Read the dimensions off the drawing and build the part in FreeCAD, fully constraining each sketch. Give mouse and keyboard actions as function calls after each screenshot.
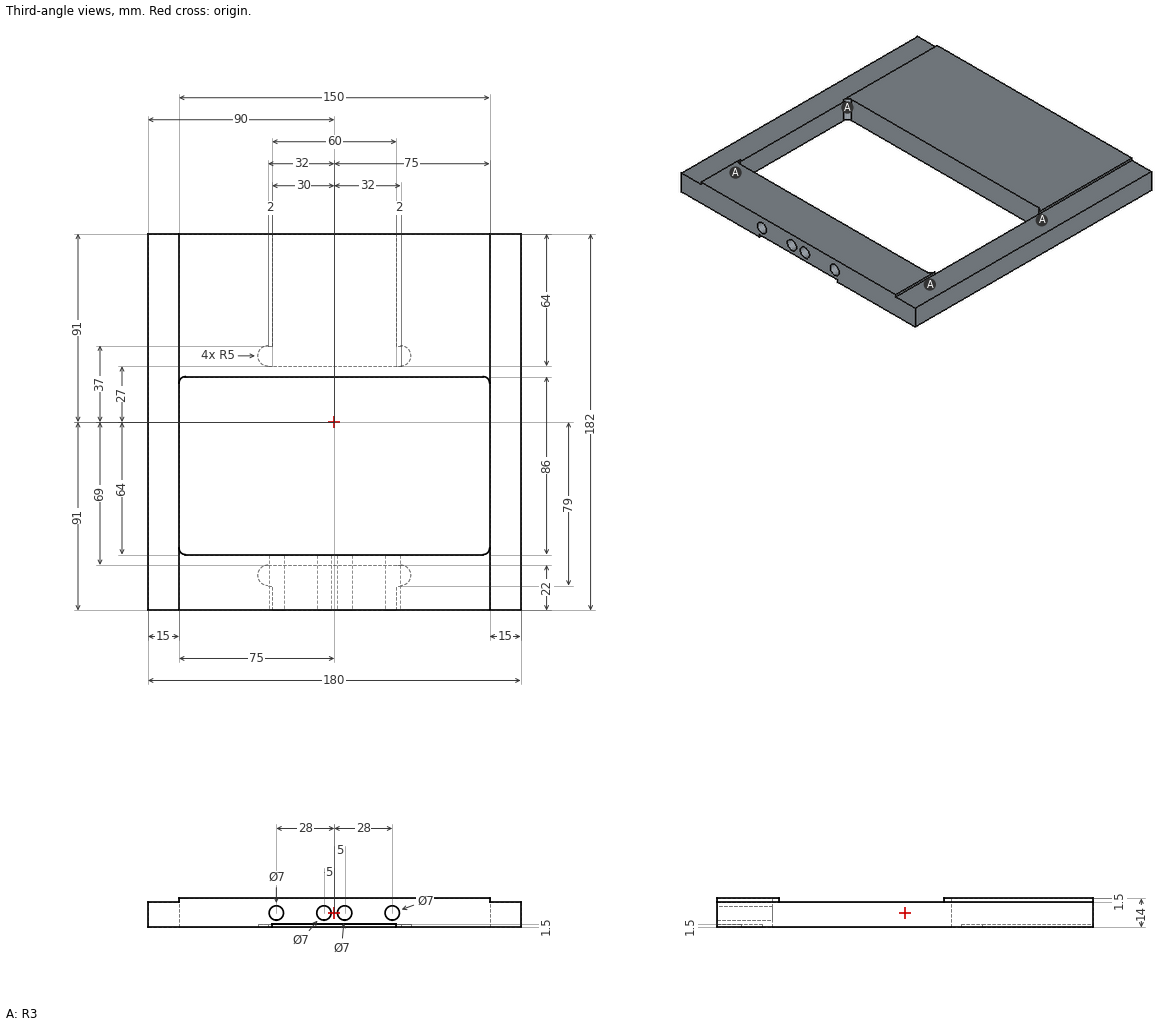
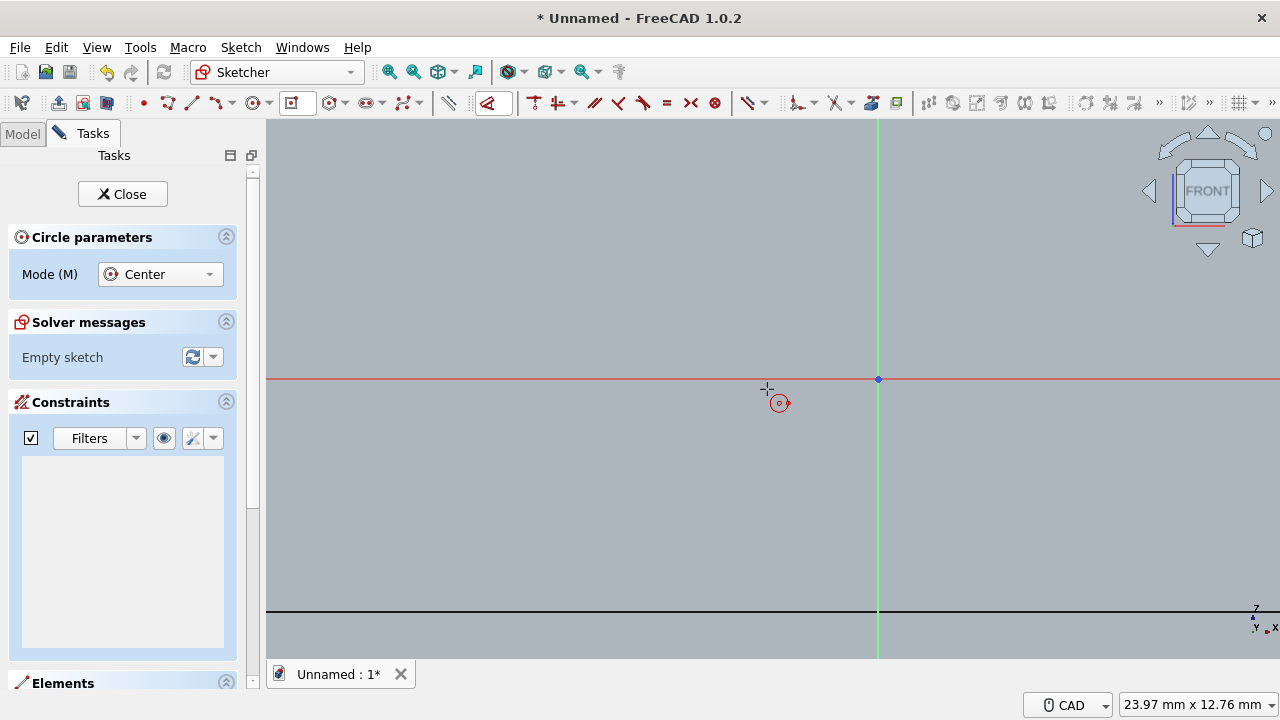
click(667, 379)
move(771, 275)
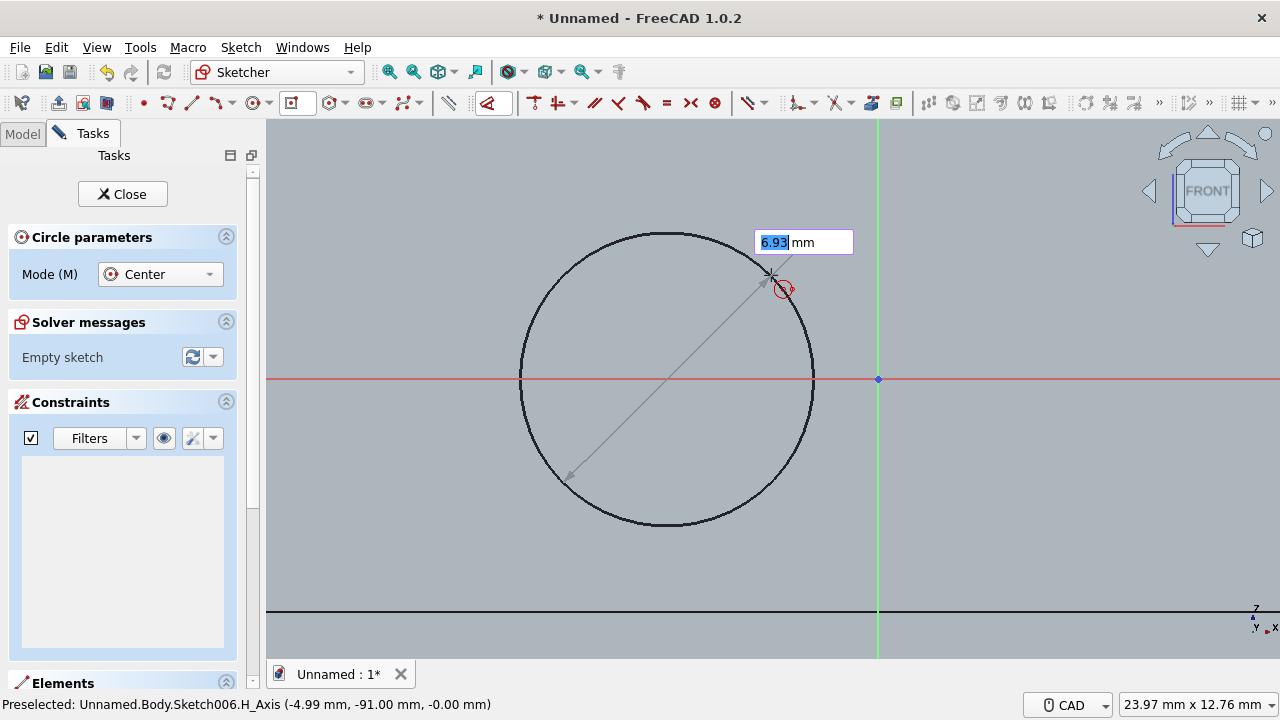
text(7)
key(Return)
key(Escape)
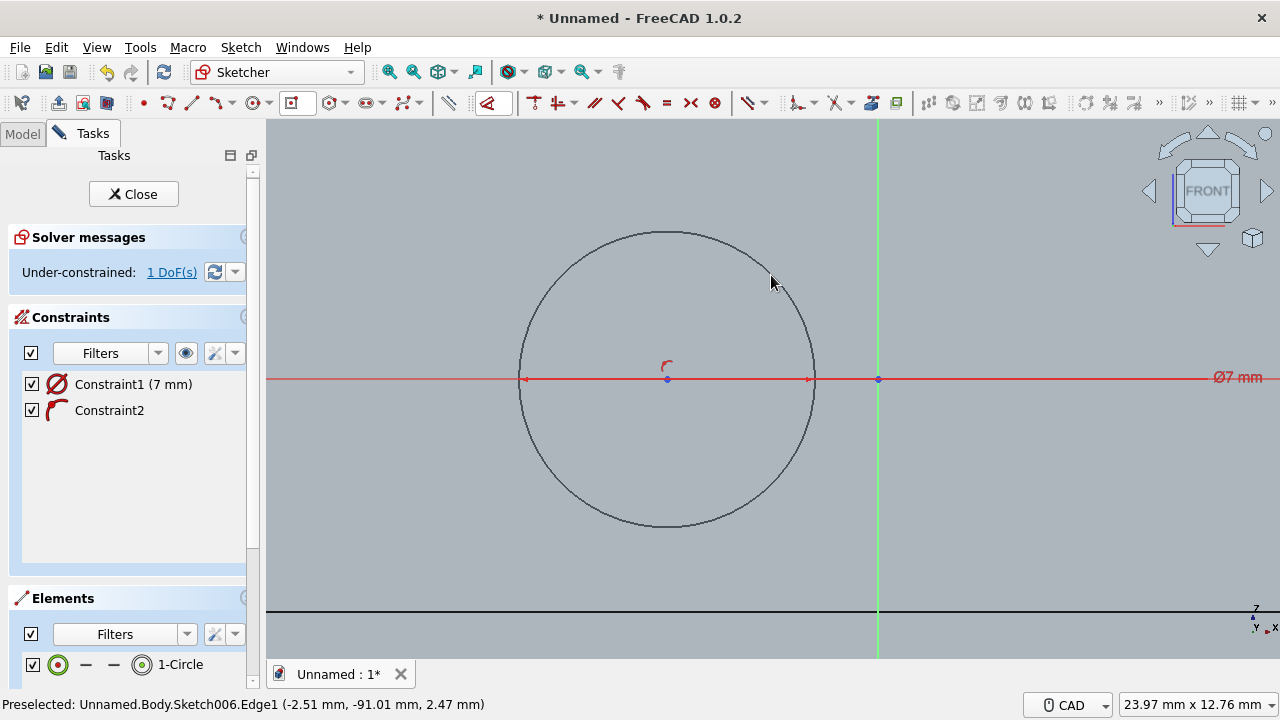
click(667, 379)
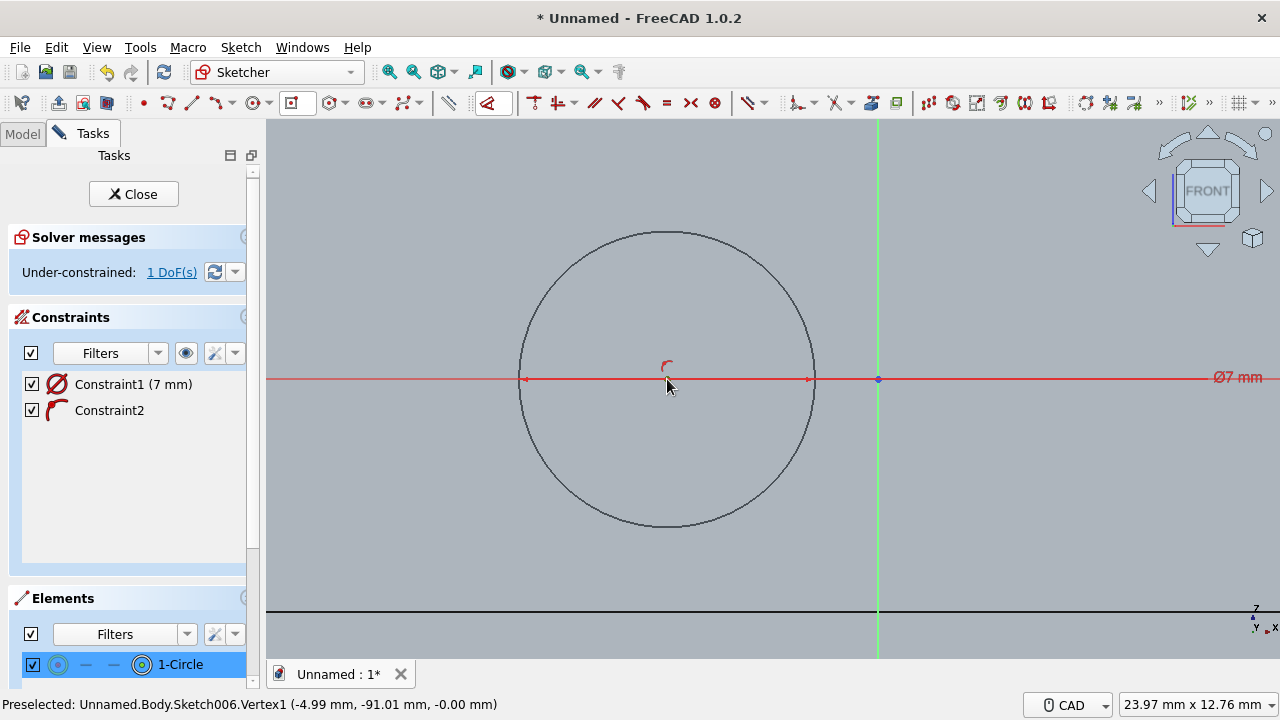
key(l)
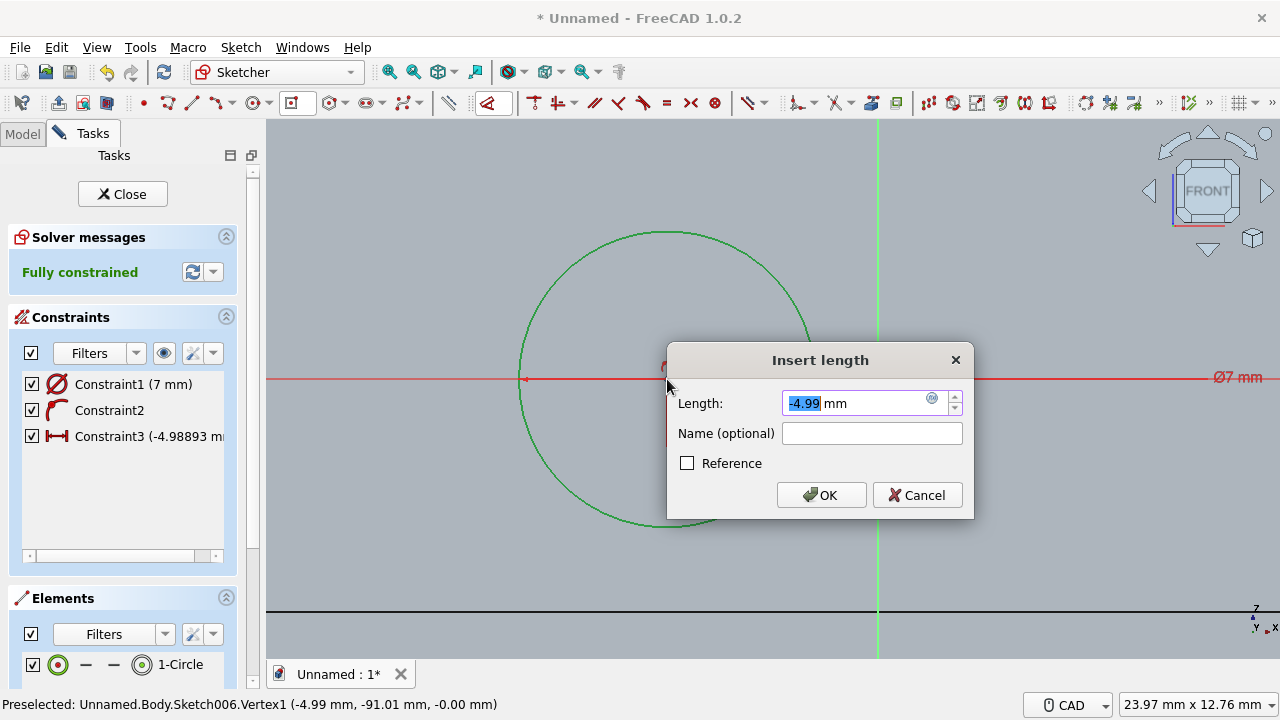
text(-5)
key(Return)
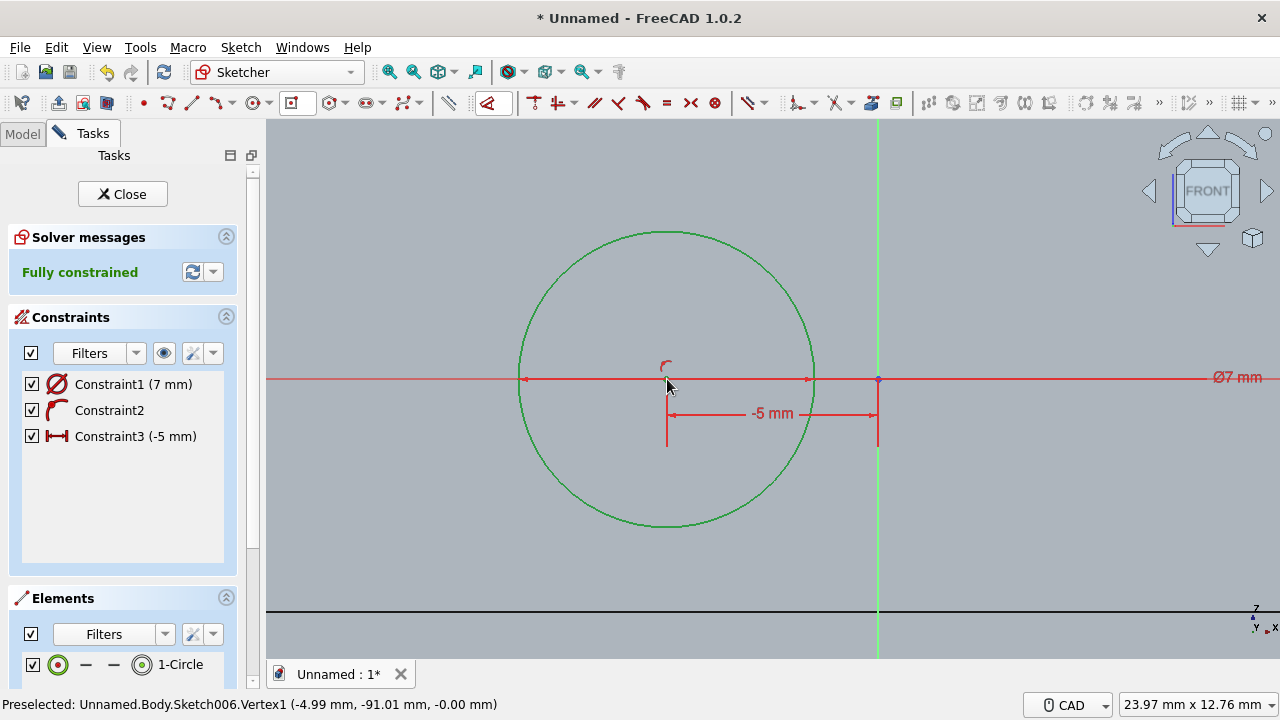
click(123, 194)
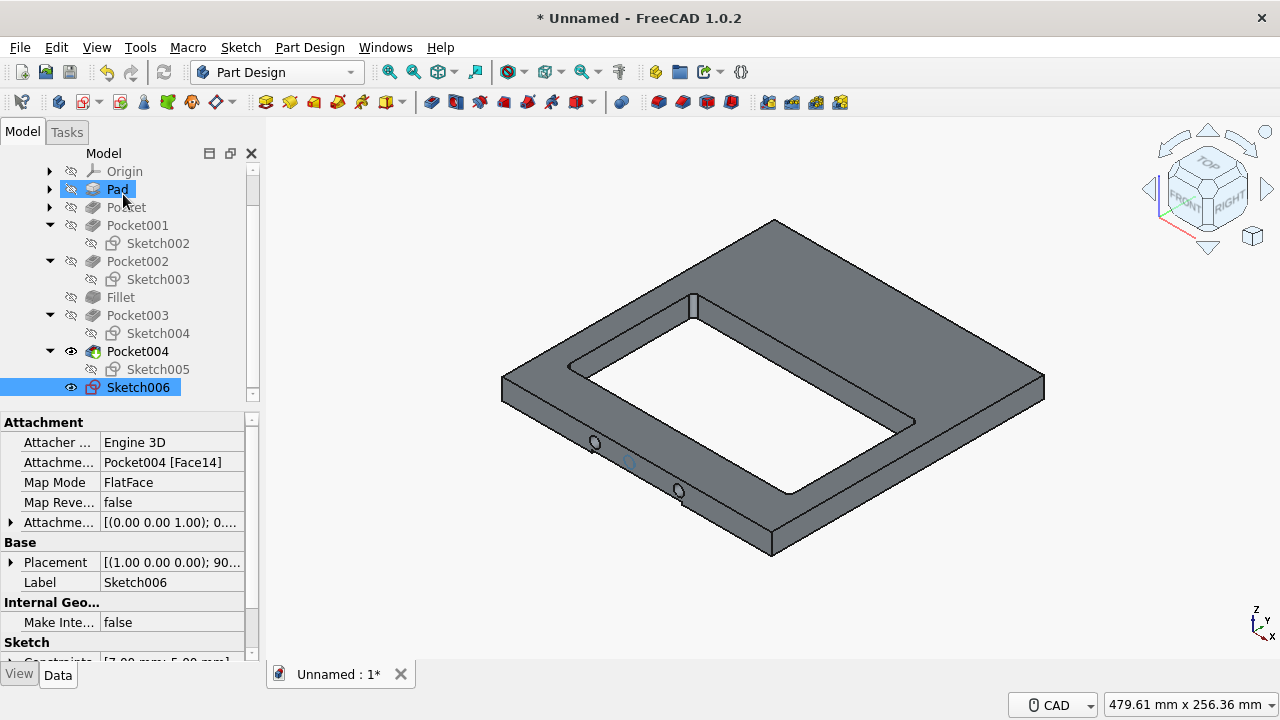
click(432, 102)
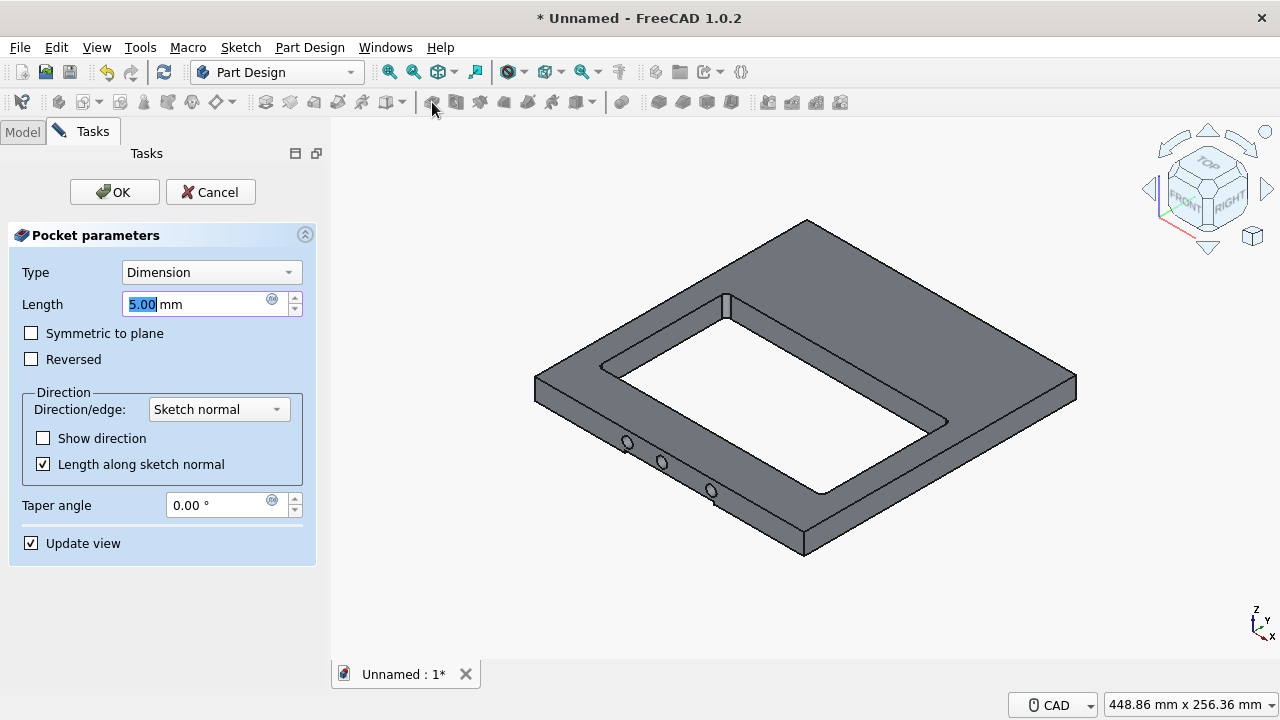
click(212, 272)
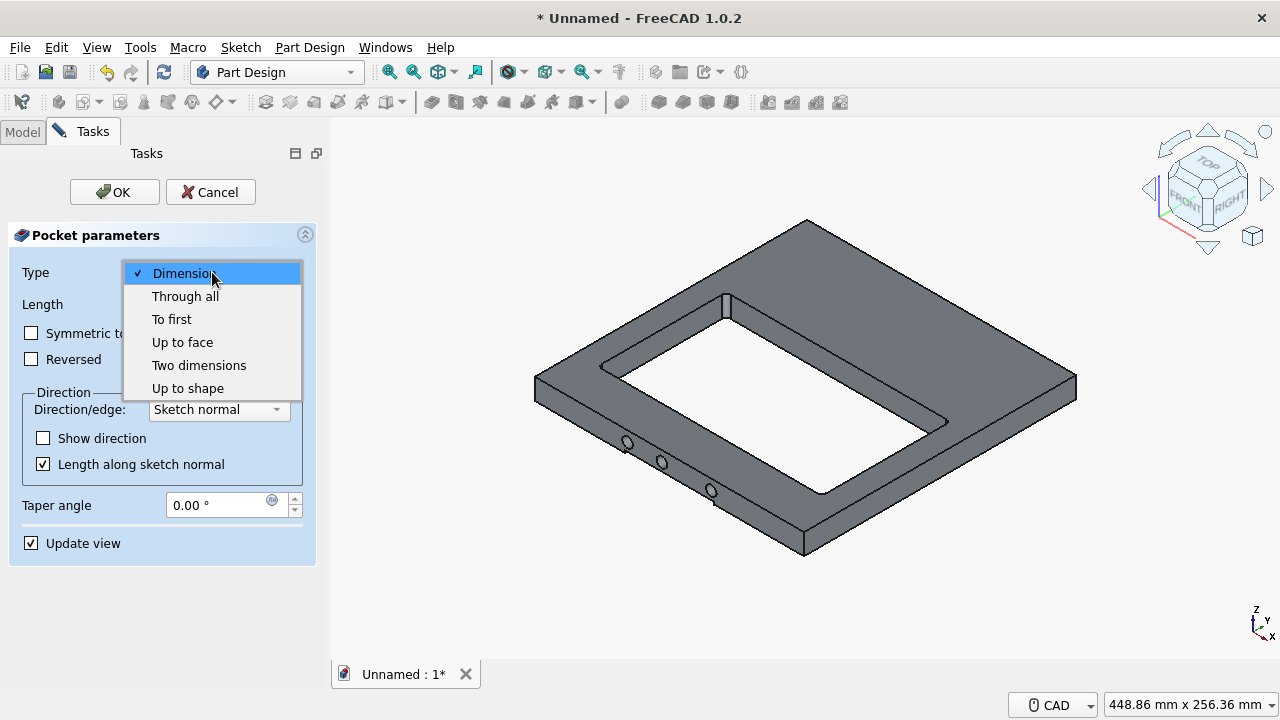
click(212, 320)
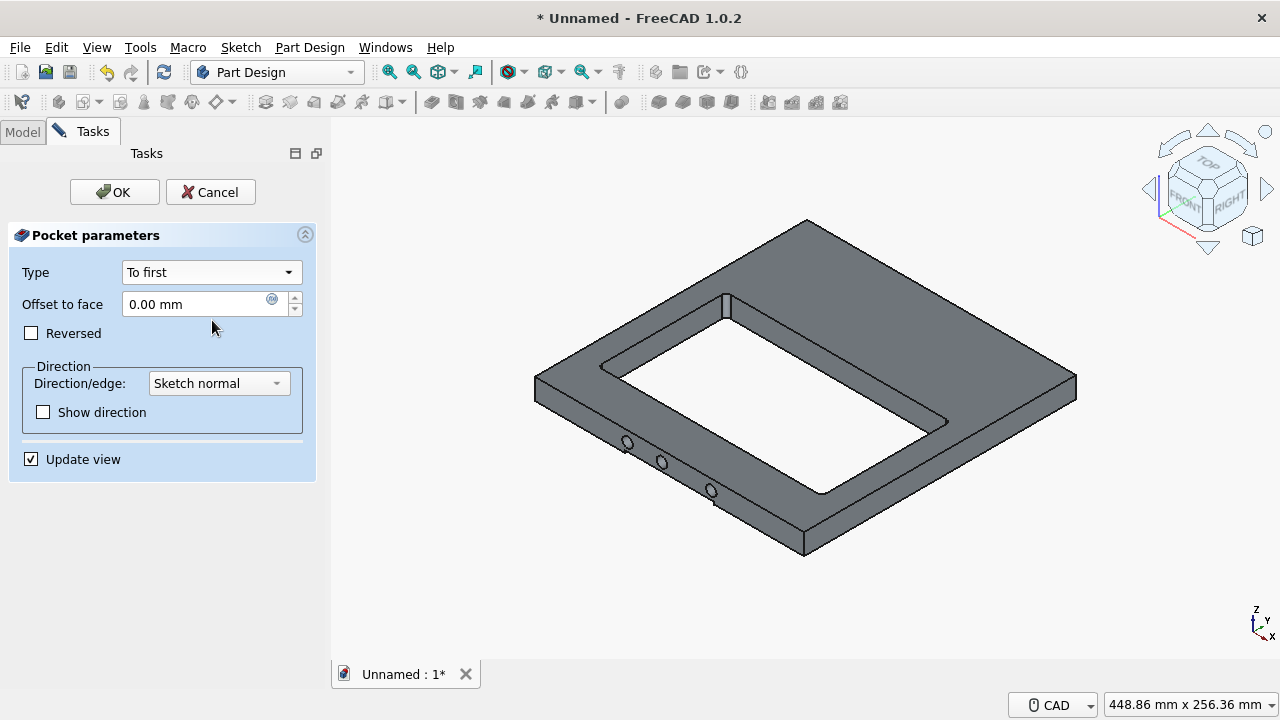
click(115, 192)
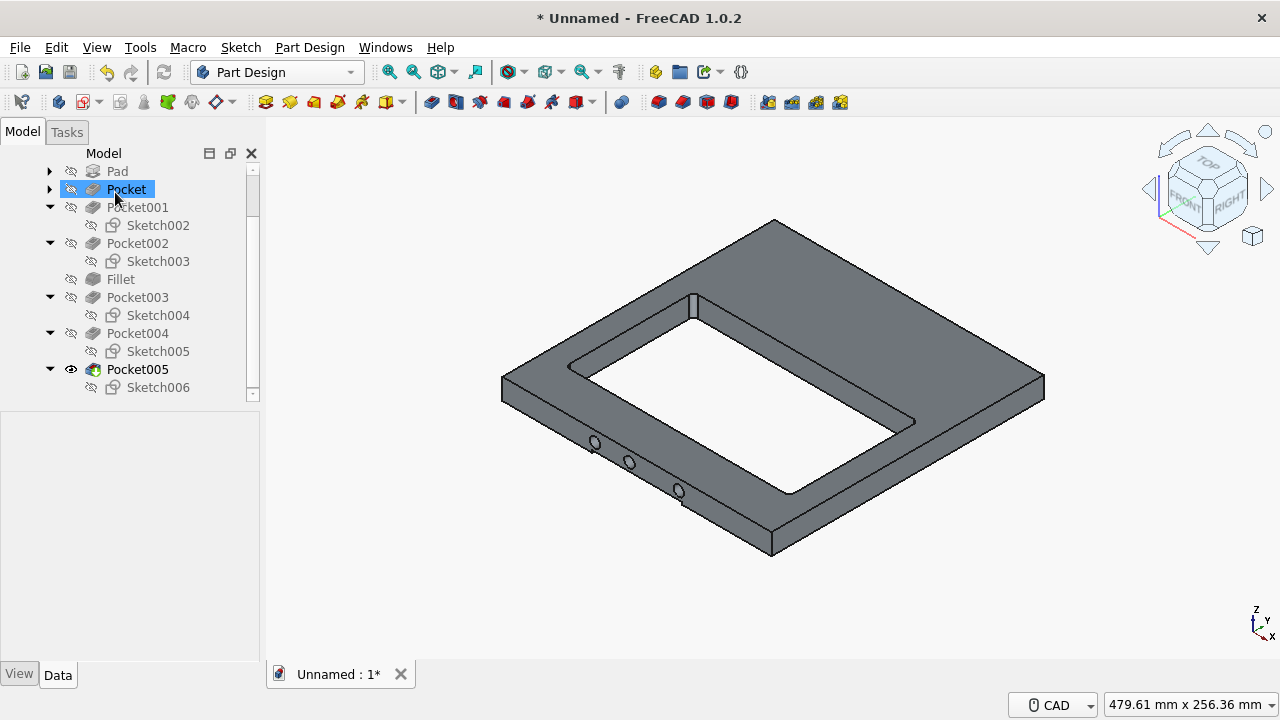
click(752, 532)